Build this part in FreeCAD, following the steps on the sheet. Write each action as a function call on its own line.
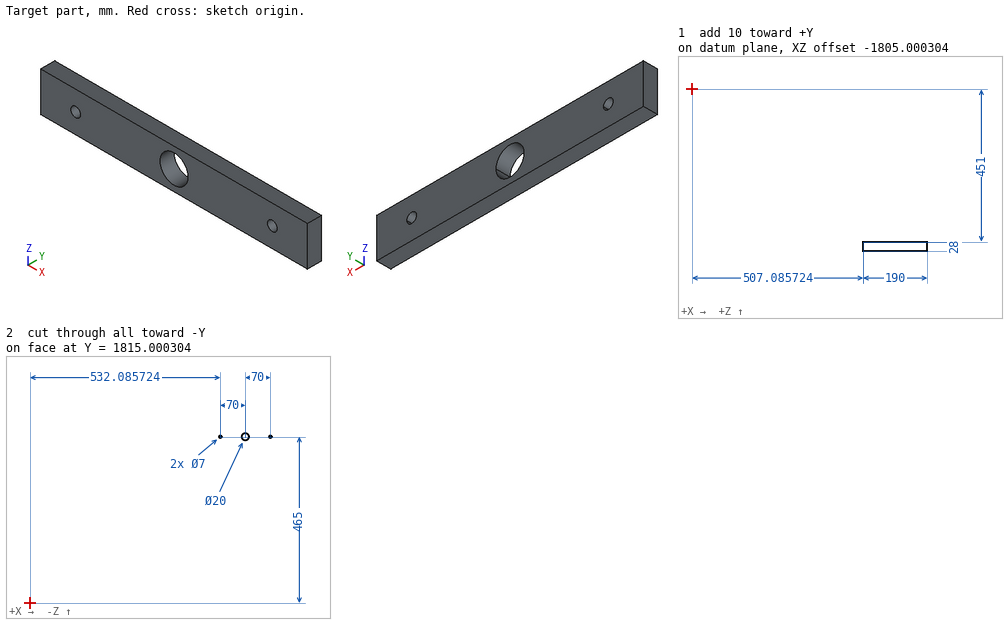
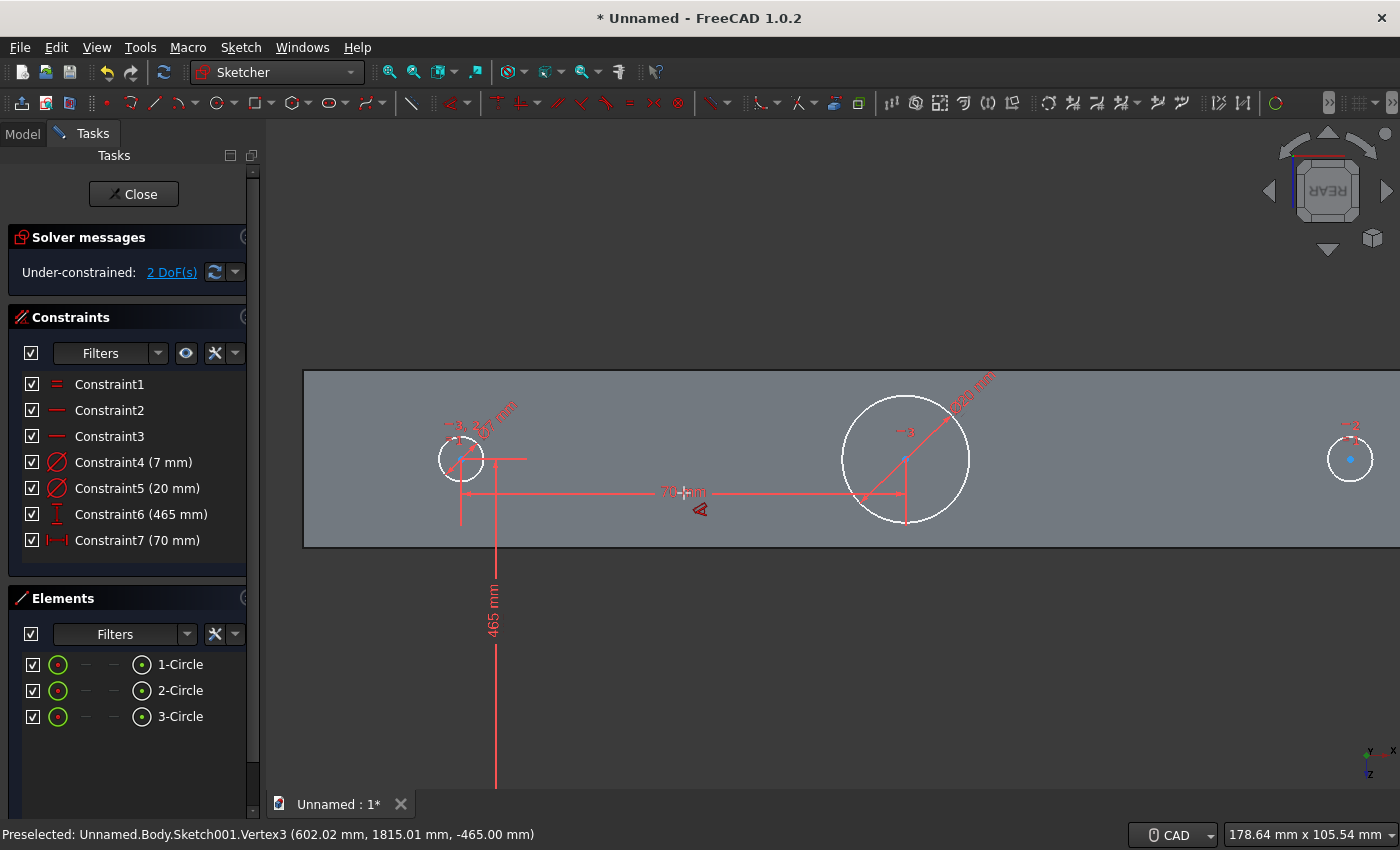
scroll(477, 443, down, 2)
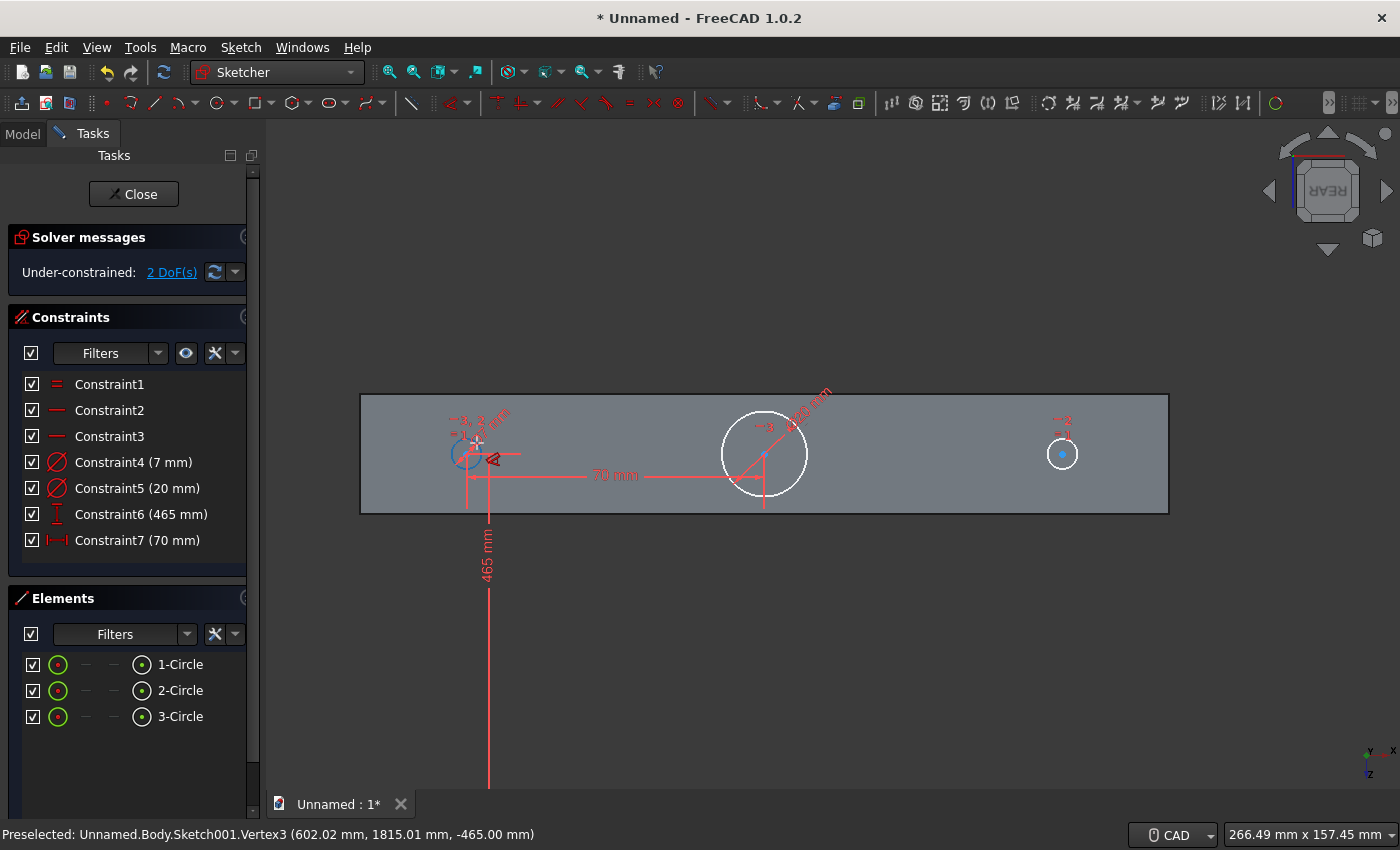
click(1062, 454)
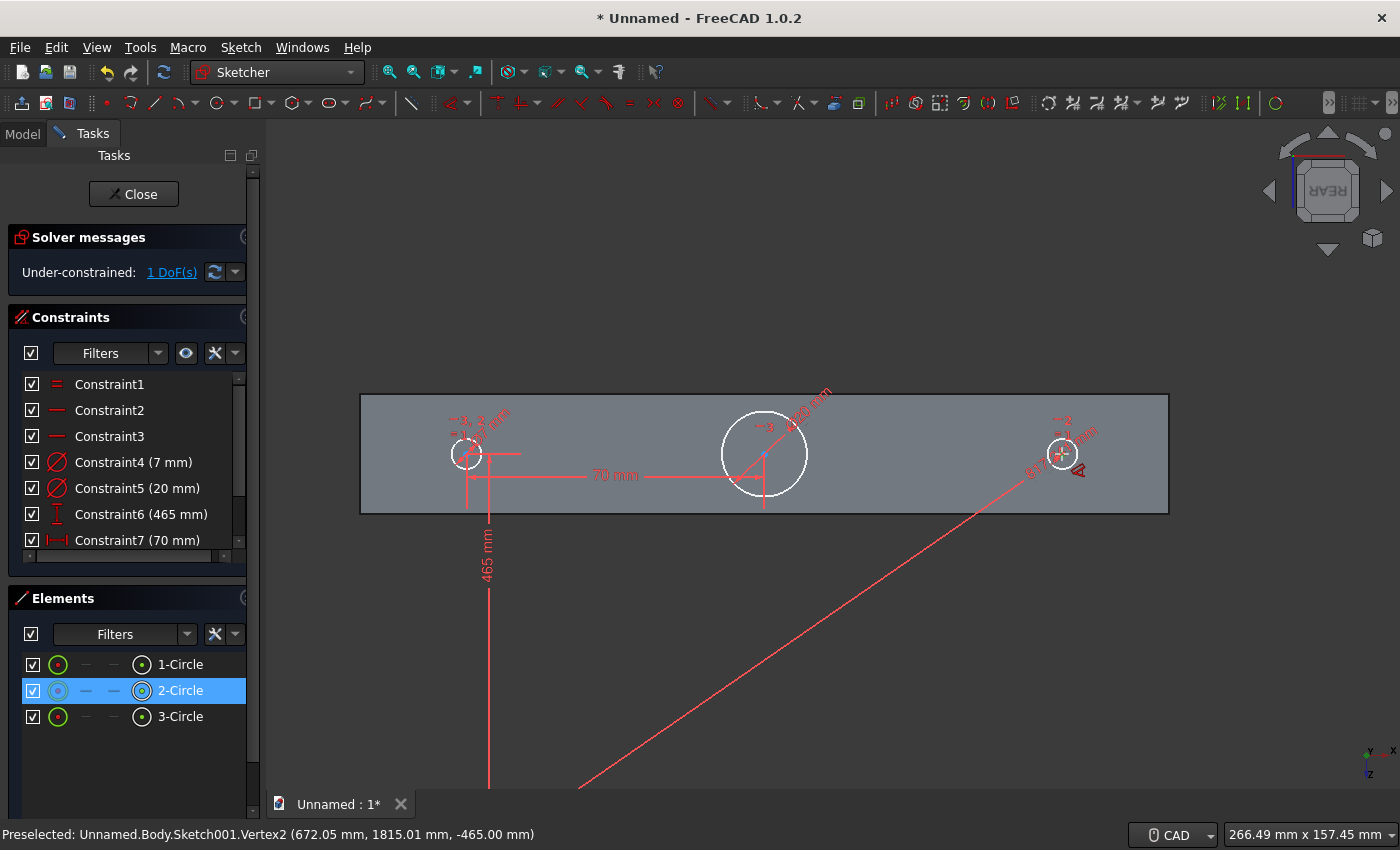
click(764, 454)
click(913, 488)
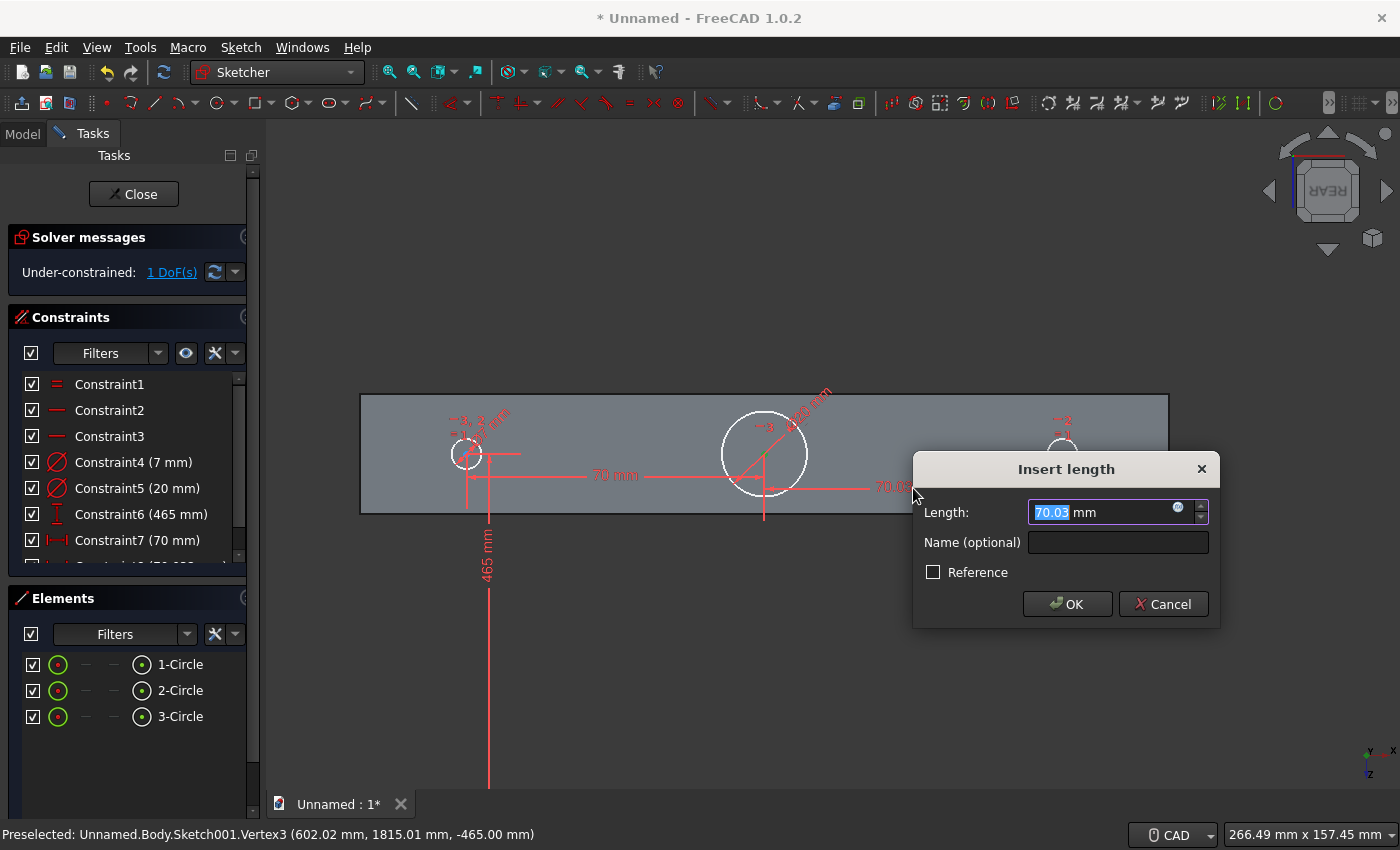
text(70)
key(Return)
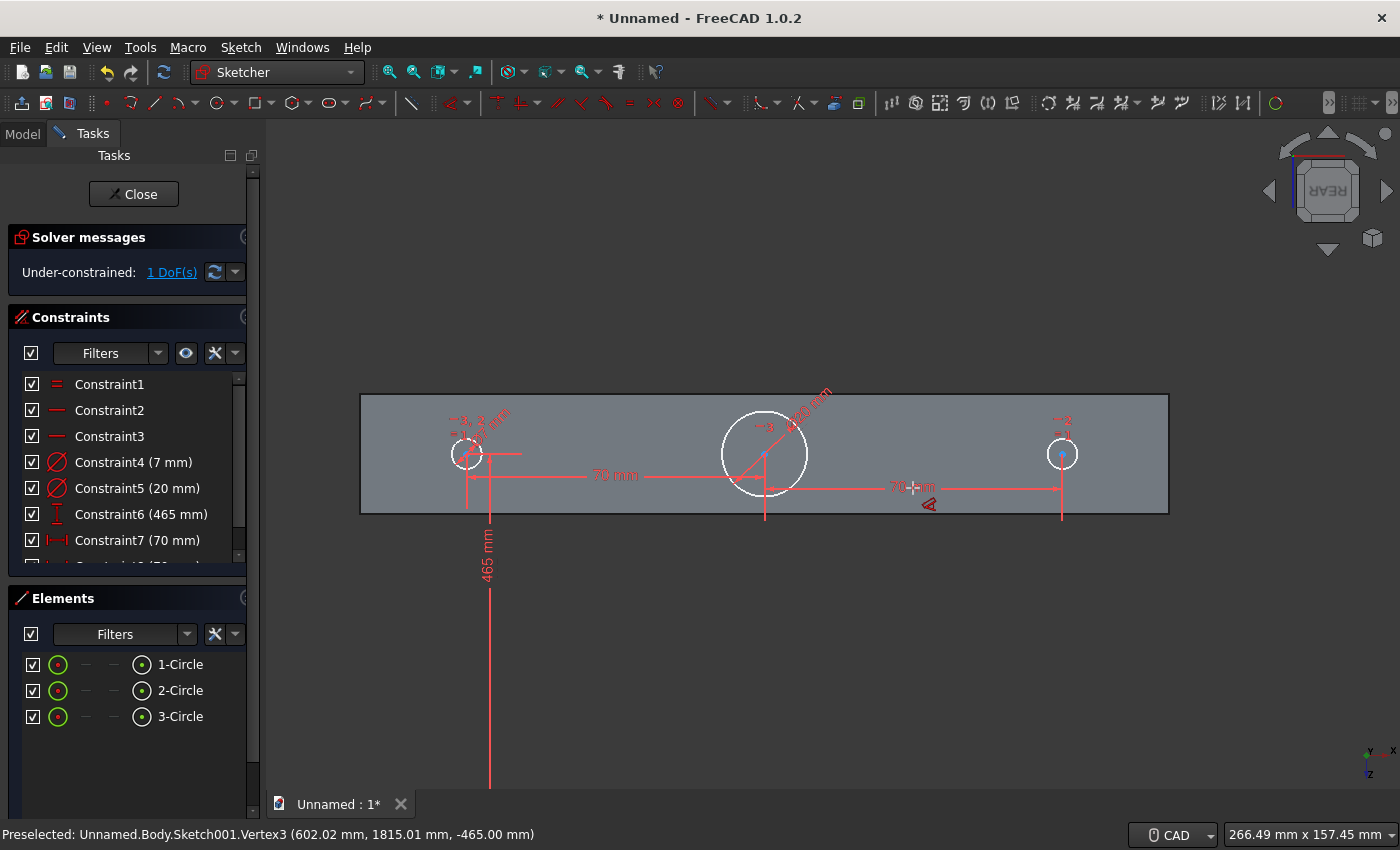
click(467, 454)
click(380, 420)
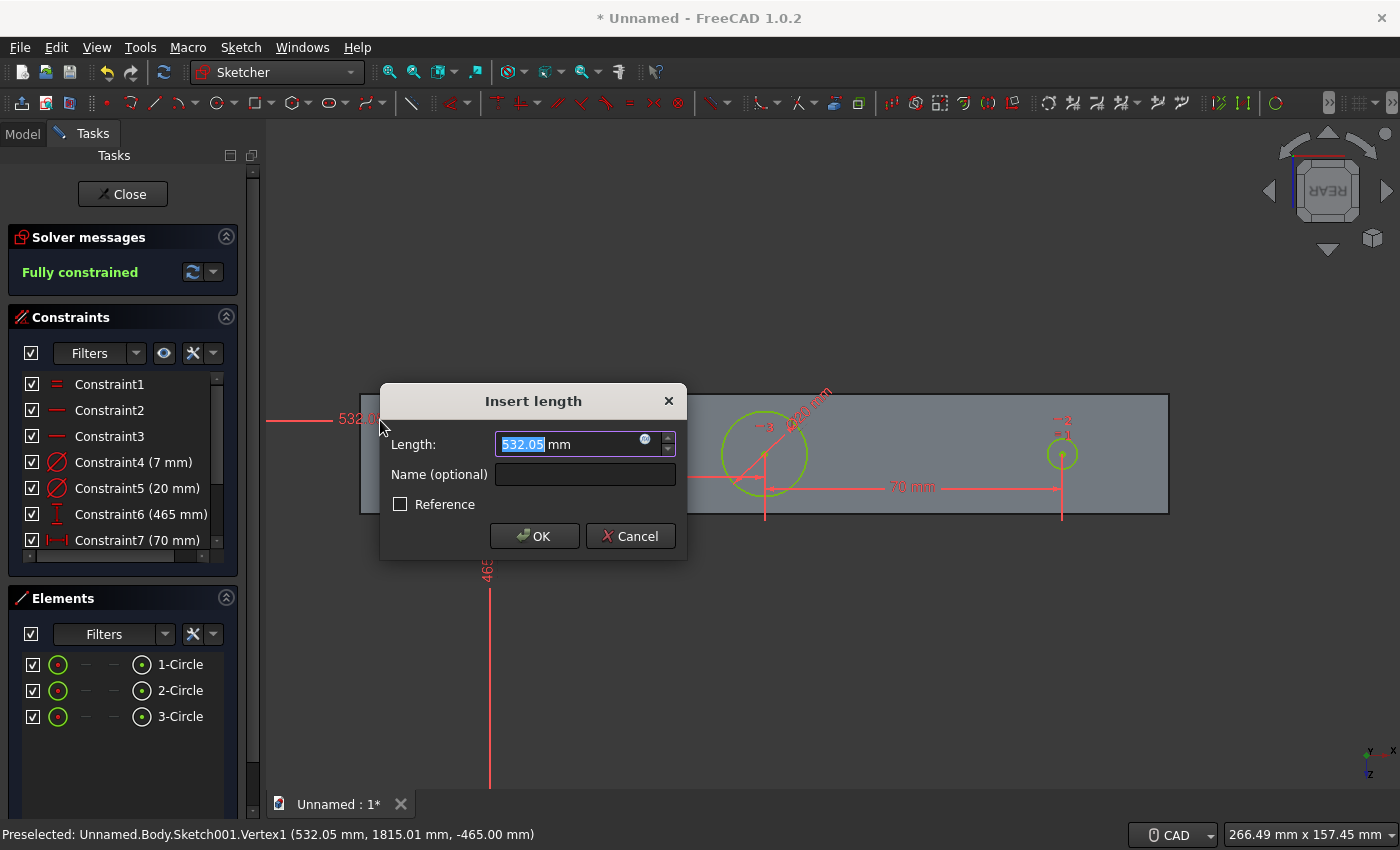
text(532.085724)
key(Return)
key(Escape)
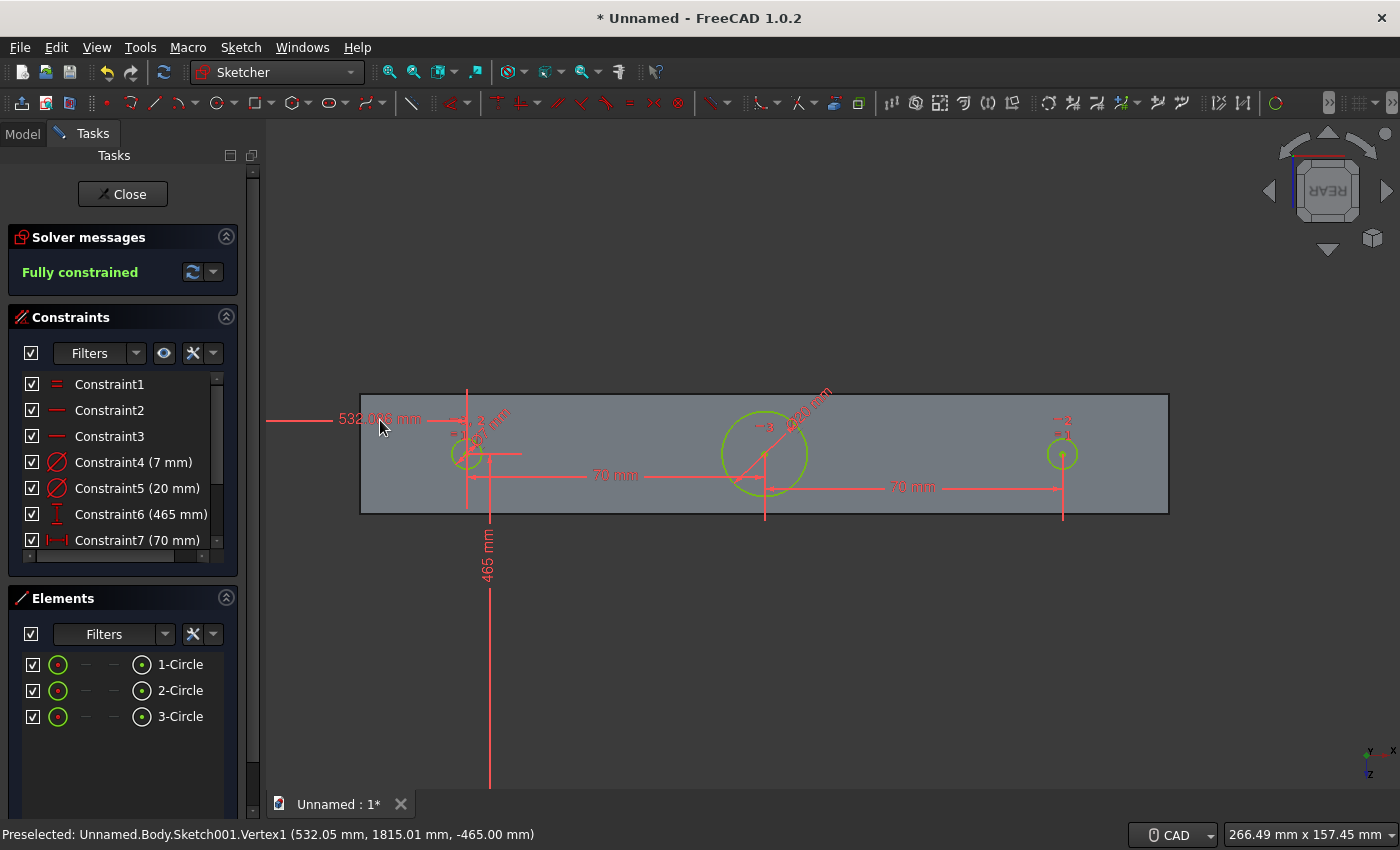
click(123, 194)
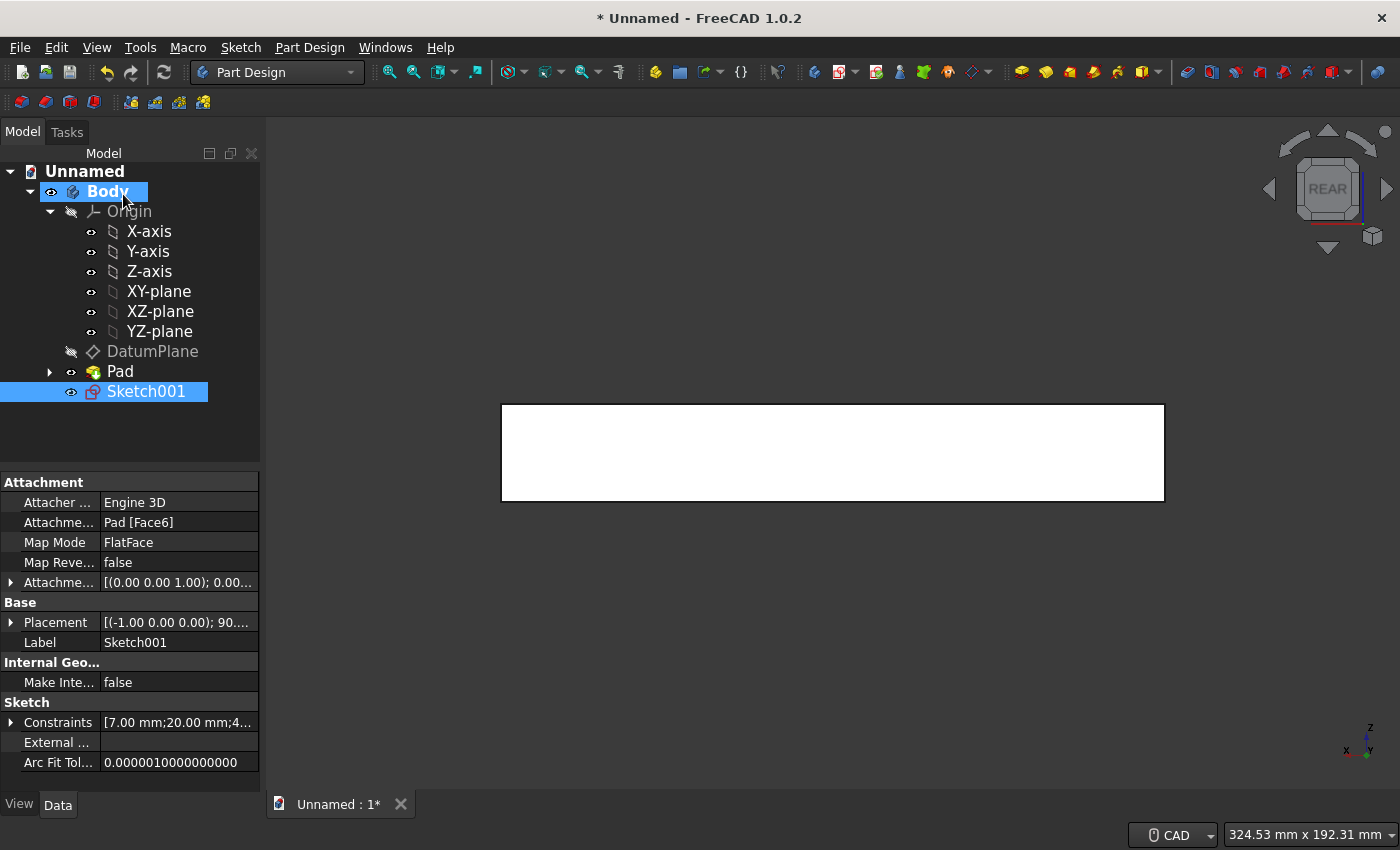
click(1188, 72)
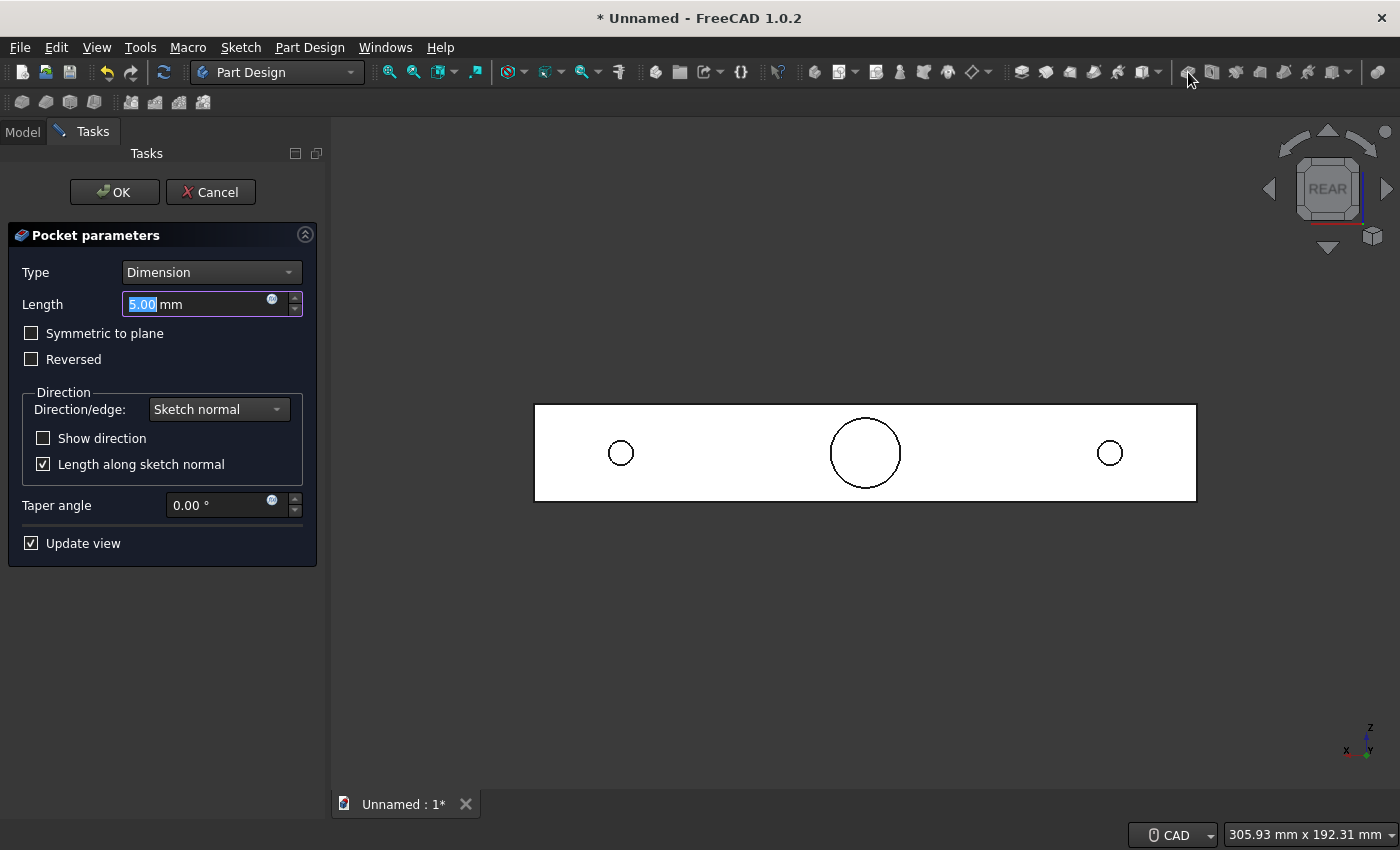
click(212, 272)